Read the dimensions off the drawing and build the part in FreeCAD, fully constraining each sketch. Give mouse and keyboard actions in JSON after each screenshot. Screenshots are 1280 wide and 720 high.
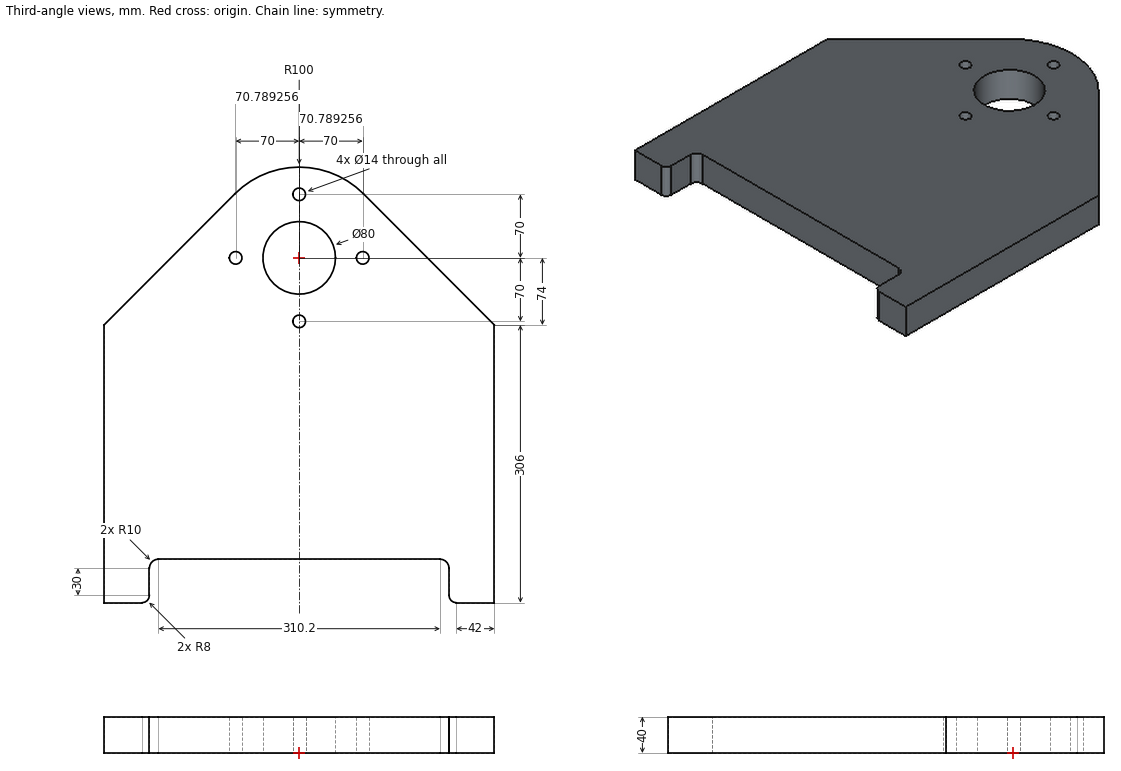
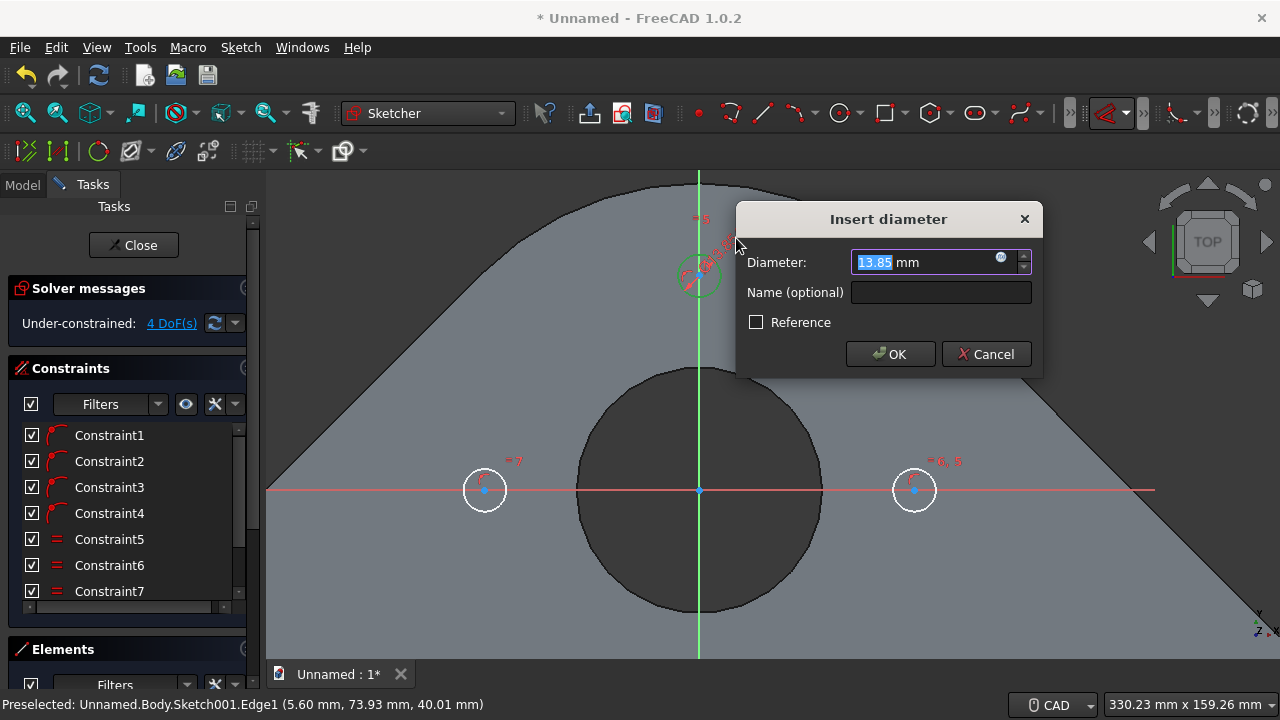
{"action": "type", "text": "14"}
{"action": "key", "text": "Return"}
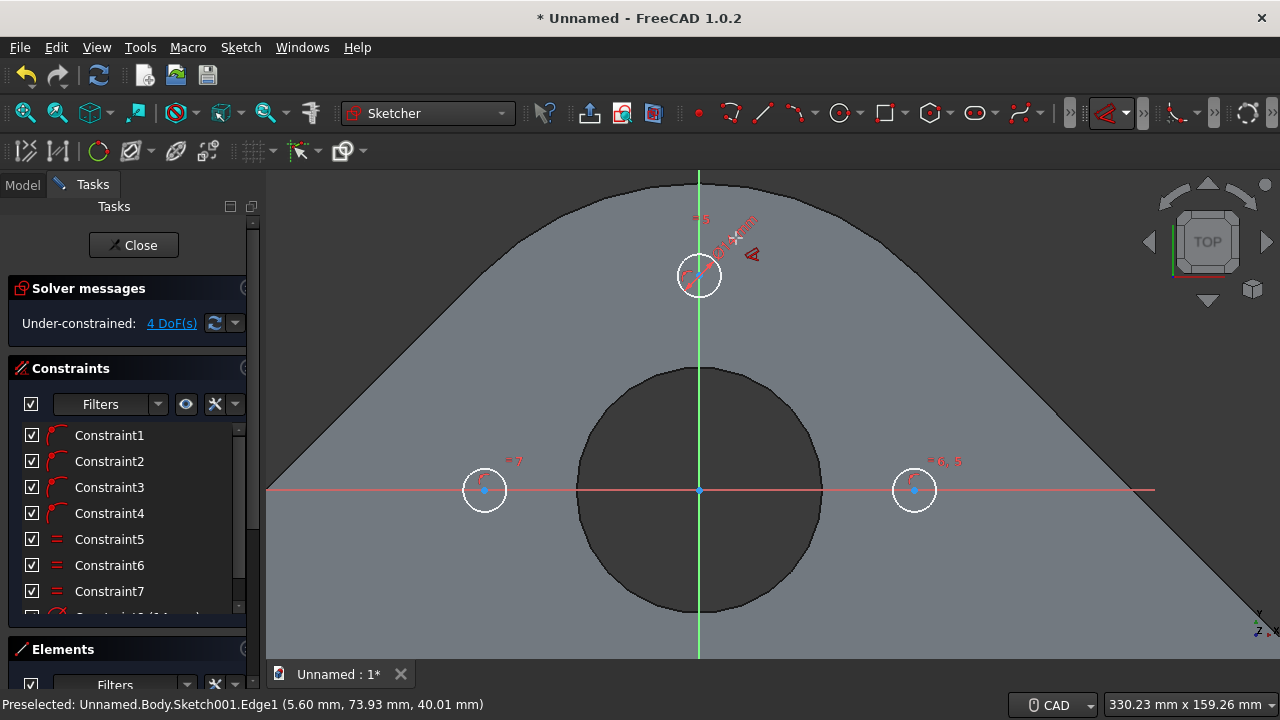
{"action": "left_click", "coordinate": [699, 276]}
{"action": "left_click", "coordinate": [733, 383]}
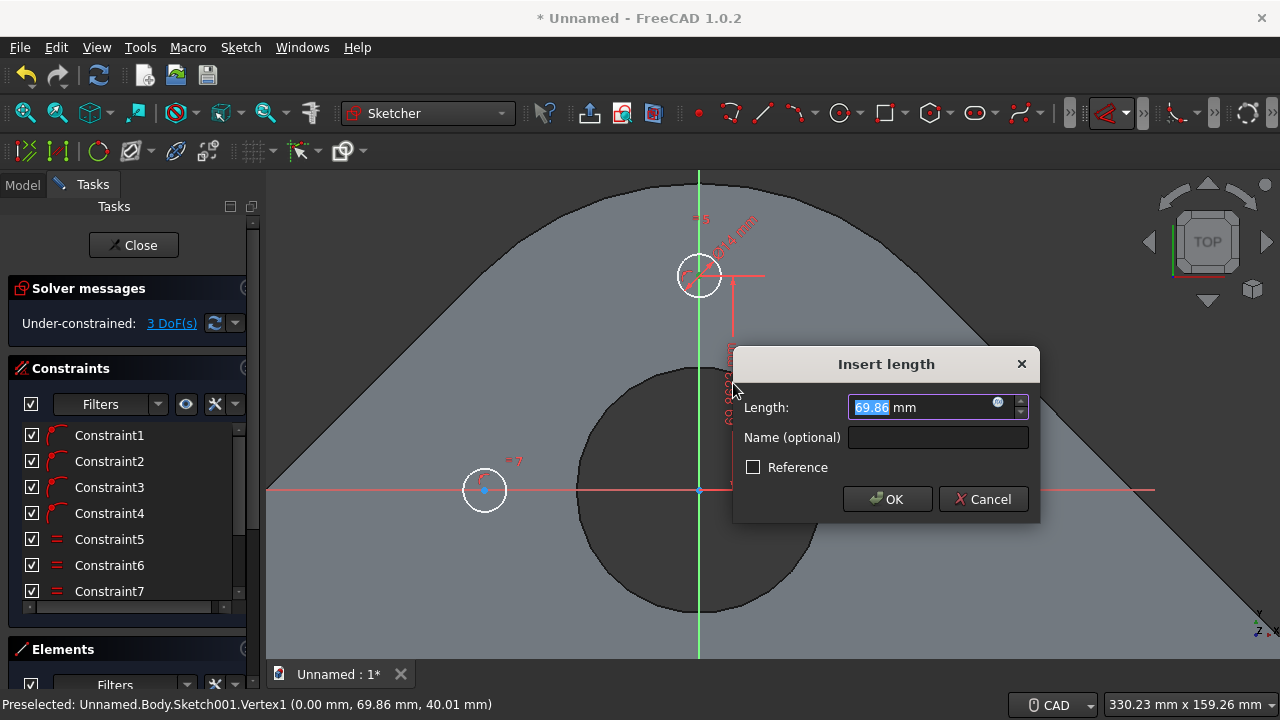
{"action": "type", "text": "70"}
{"action": "key", "text": "Return"}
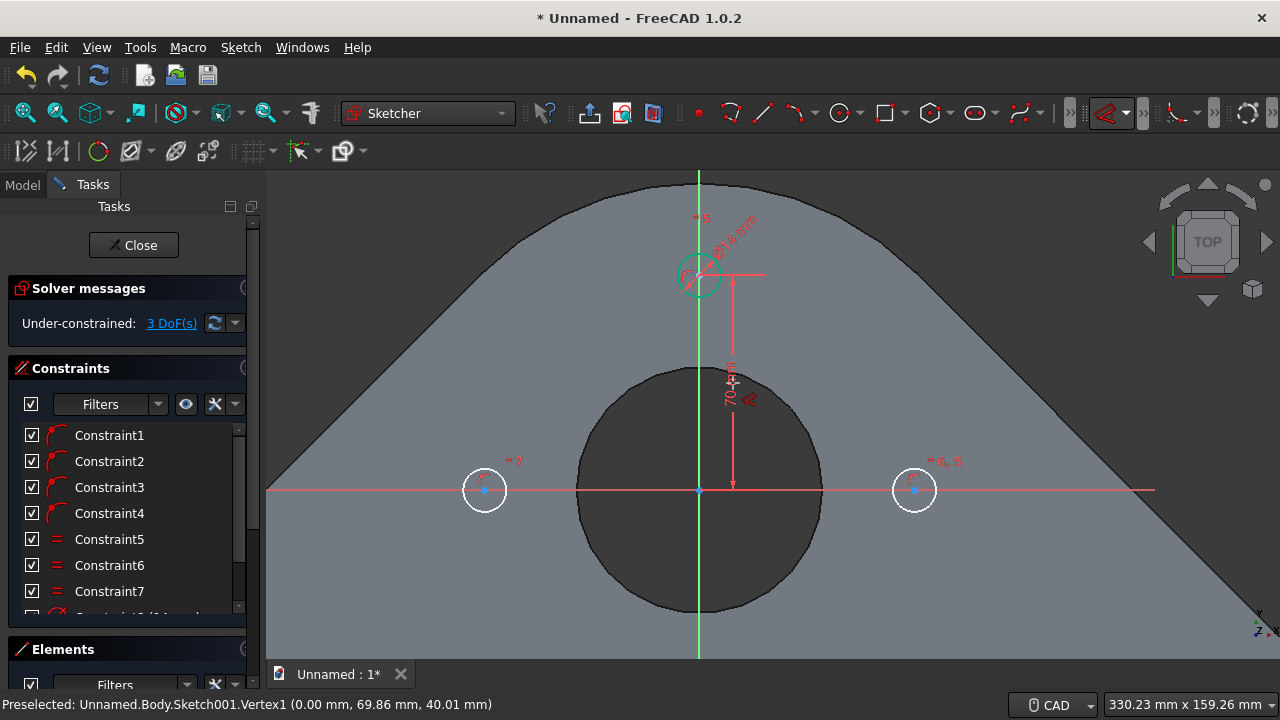
{"action": "left_click", "coordinate": [915, 490]}
{"action": "left_click", "coordinate": [807, 524]}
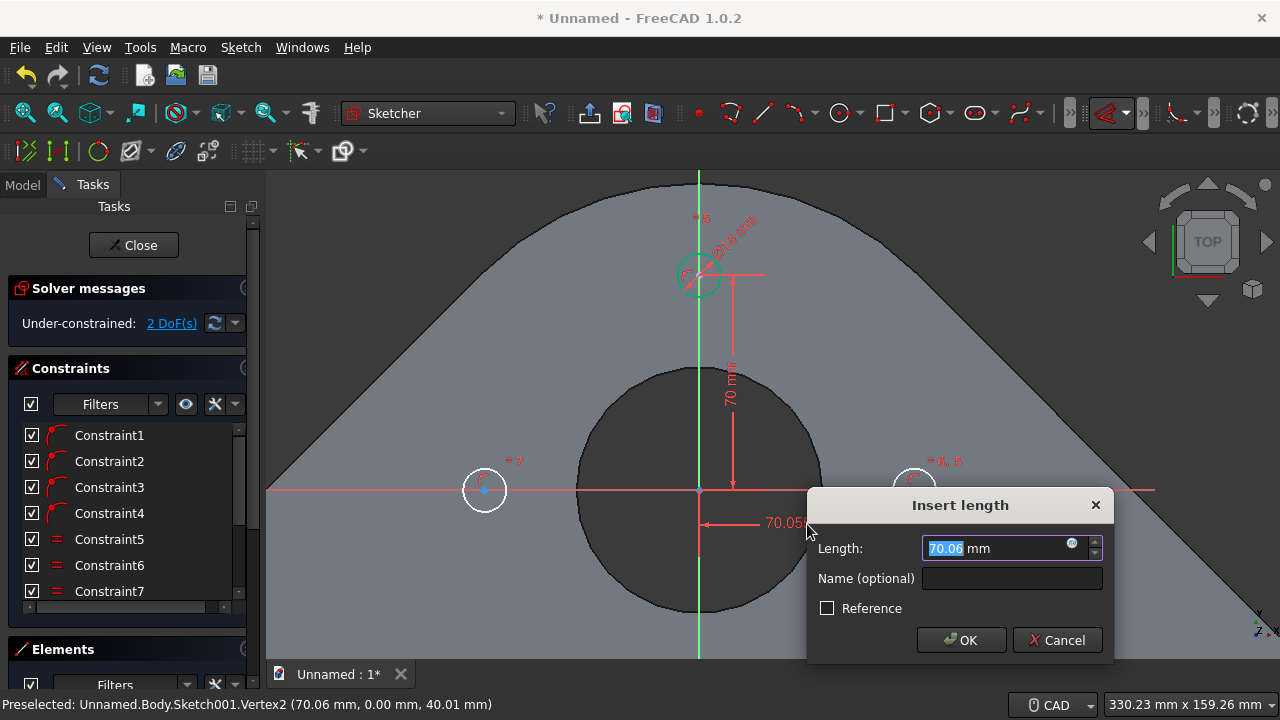
{"action": "type", "text": "70"}
{"action": "key", "text": "Return"}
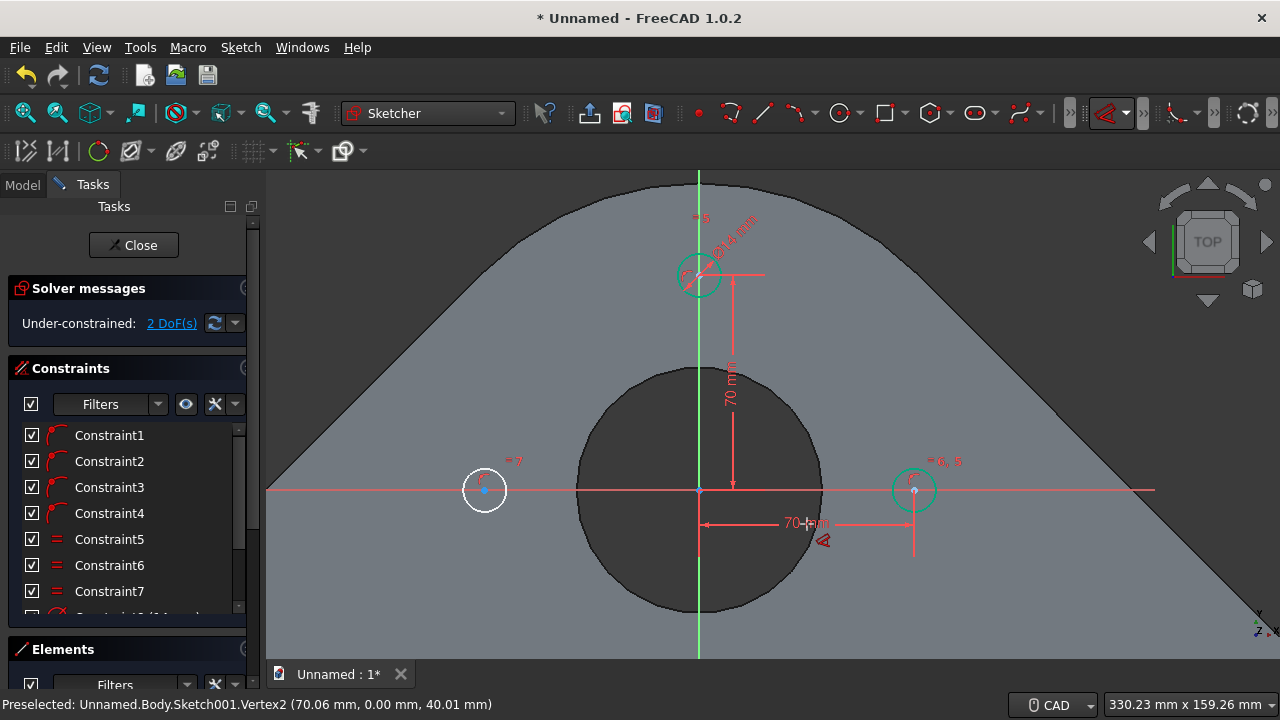
{"action": "scroll", "coordinate": [715, 260], "scroll_direction": "down", "scroll_amount": 2}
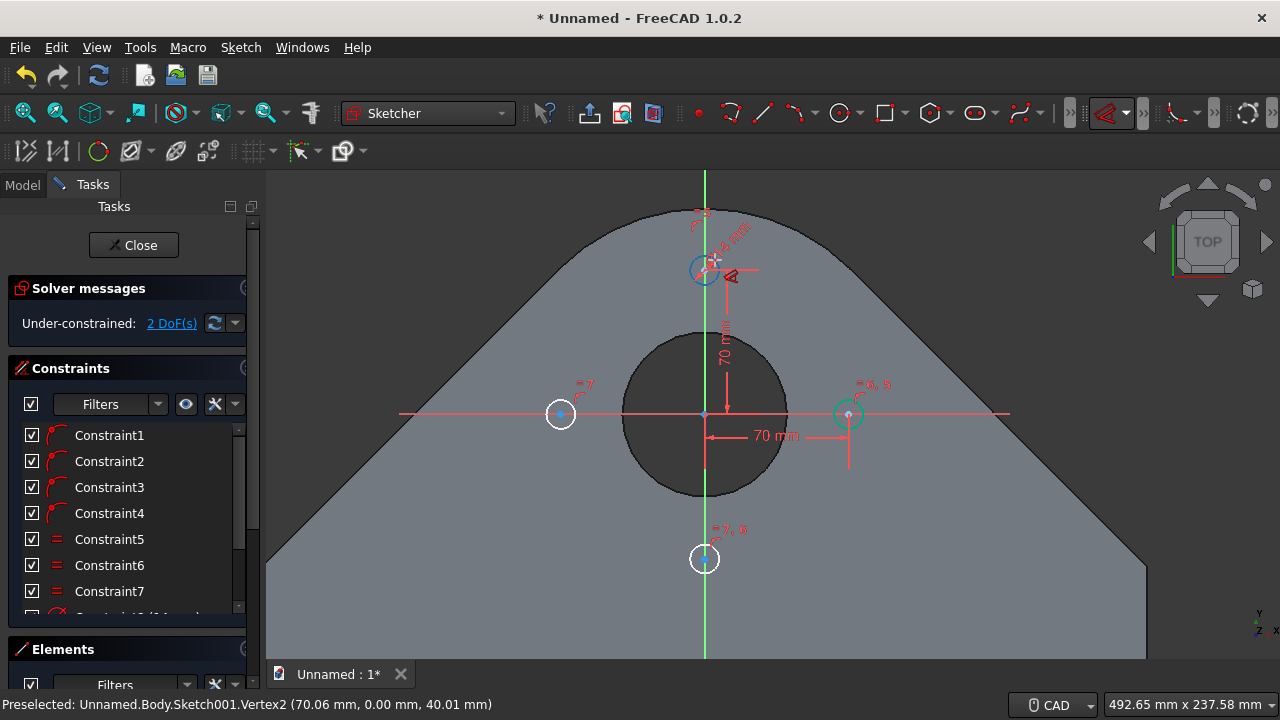
{"action": "left_click", "coordinate": [705, 559]}
{"action": "left_click", "coordinate": [739, 487]}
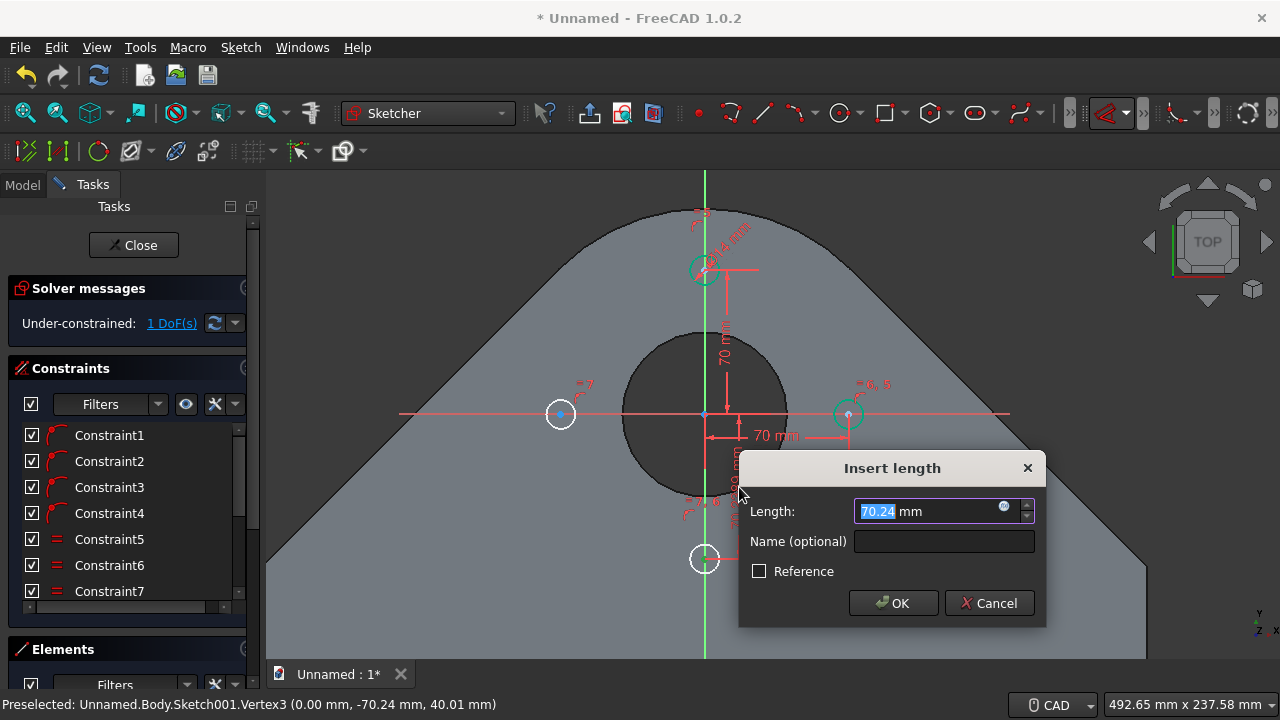
{"action": "type", "text": "70"}
{"action": "key", "text": "Return"}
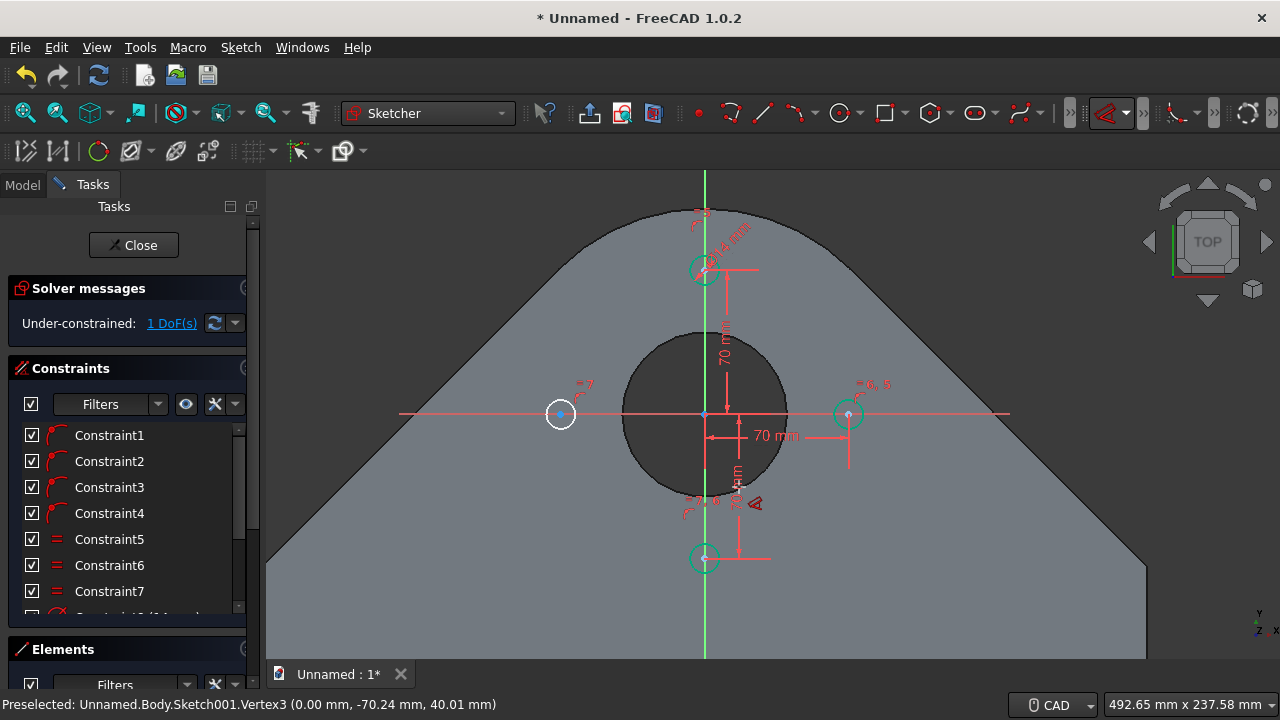
{"action": "left_click", "coordinate": [561, 414]}
{"action": "left_click", "coordinate": [633, 448]}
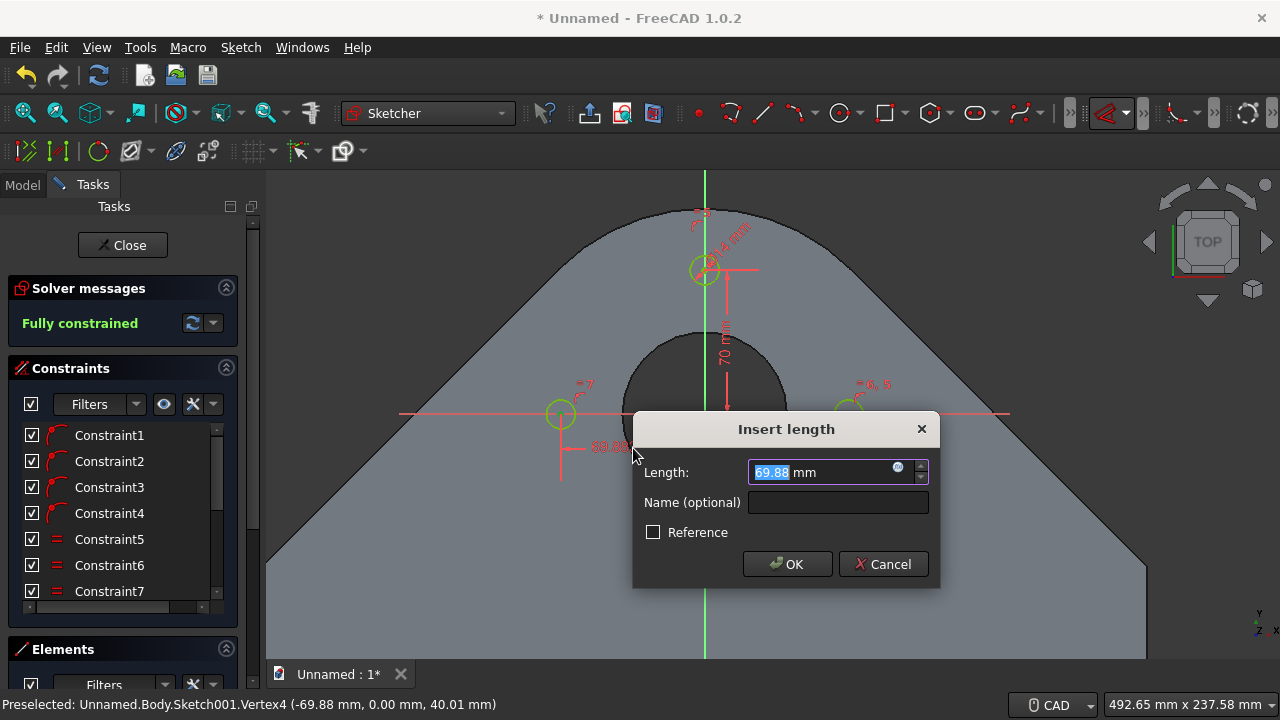
{"action": "type", "text": "70"}
{"action": "key", "text": "Return"}
{"action": "key", "text": "Escape"}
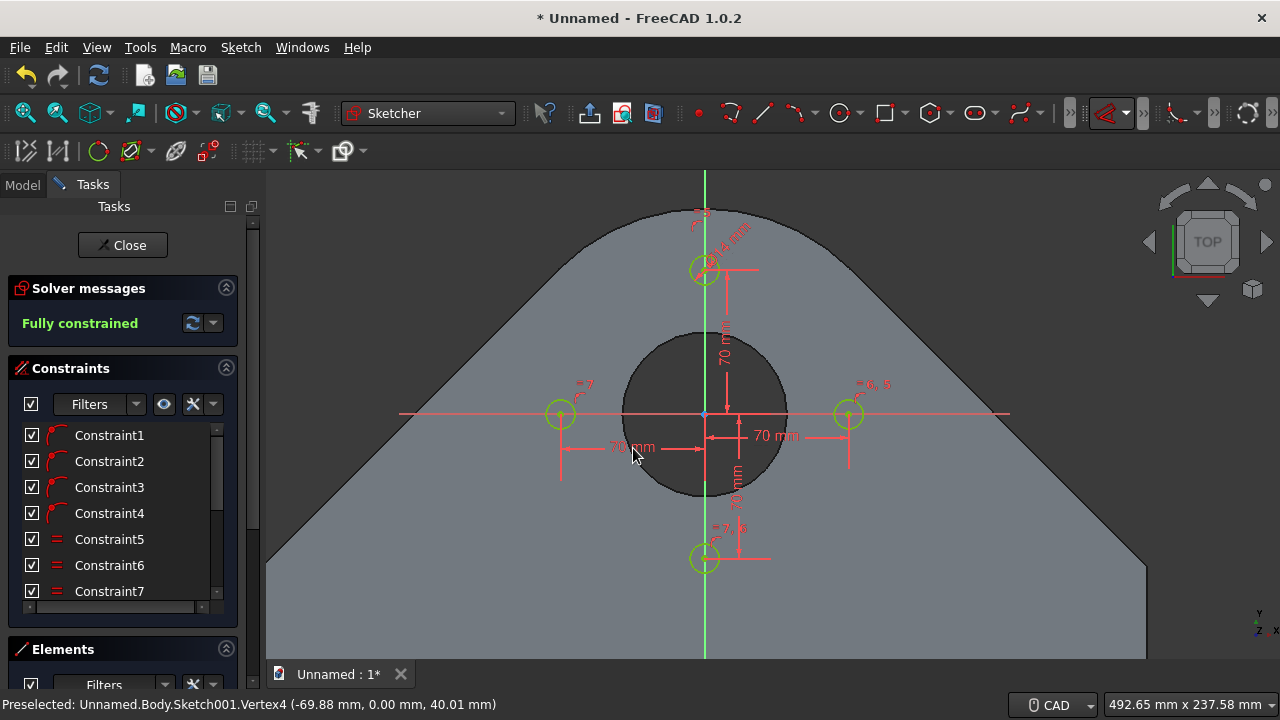
{"action": "left_click", "coordinate": [123, 245]}